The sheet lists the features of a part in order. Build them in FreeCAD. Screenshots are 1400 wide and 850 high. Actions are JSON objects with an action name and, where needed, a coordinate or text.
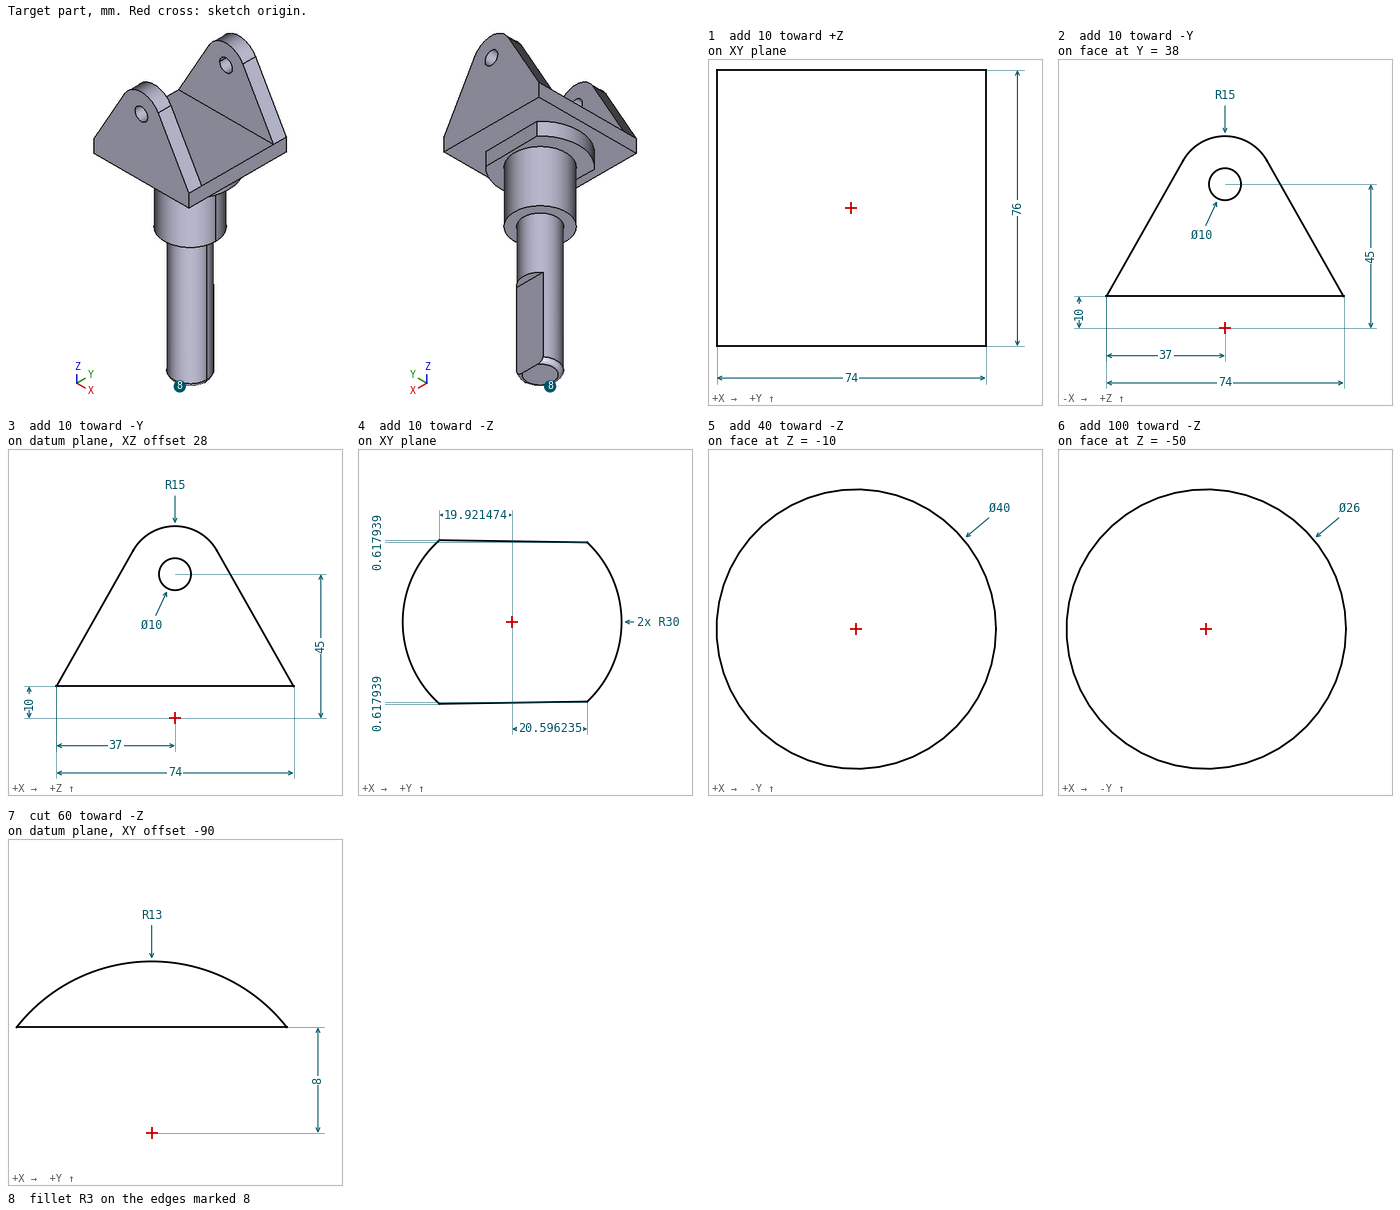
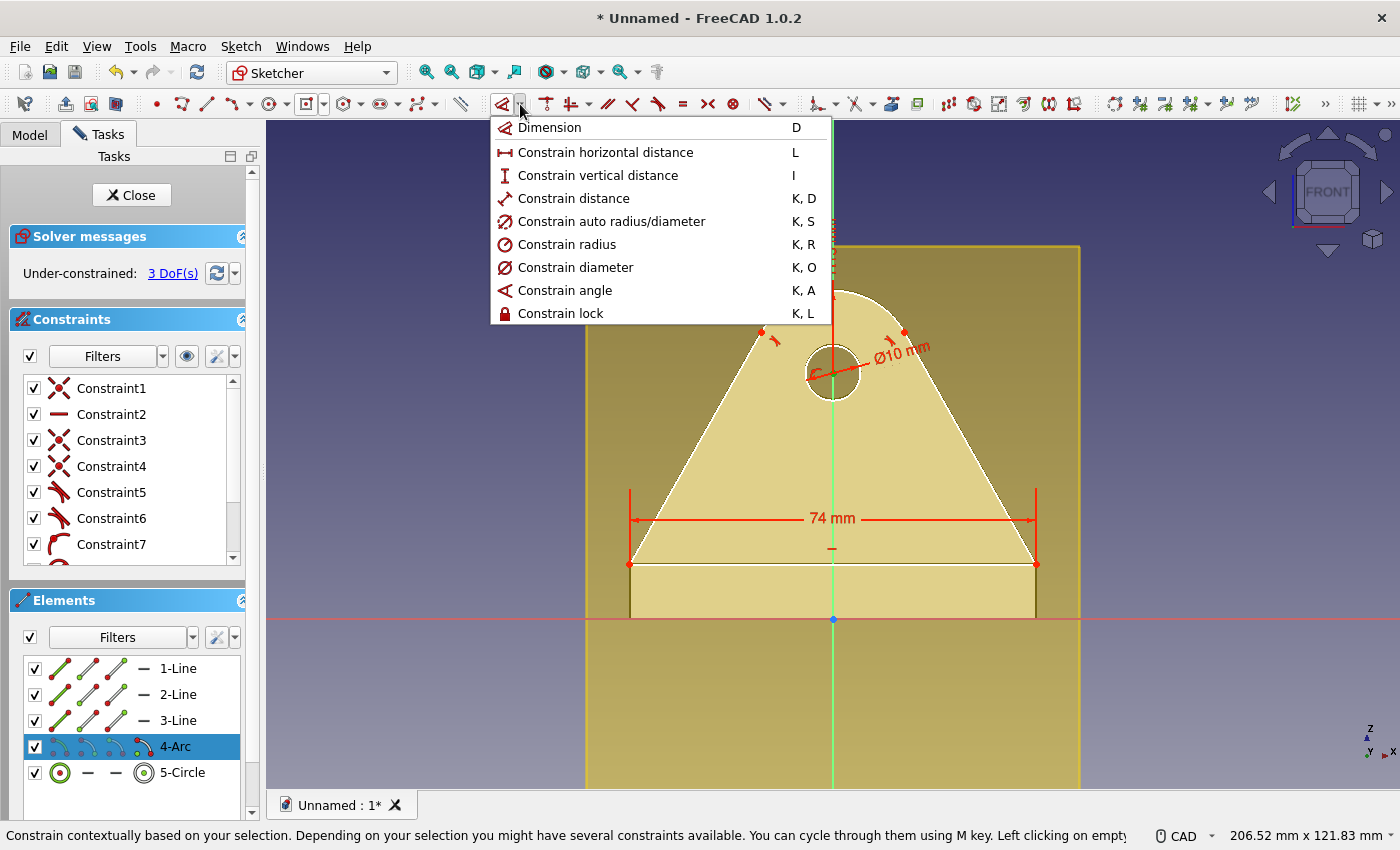
{"action": "left_click", "coordinate": [661, 176]}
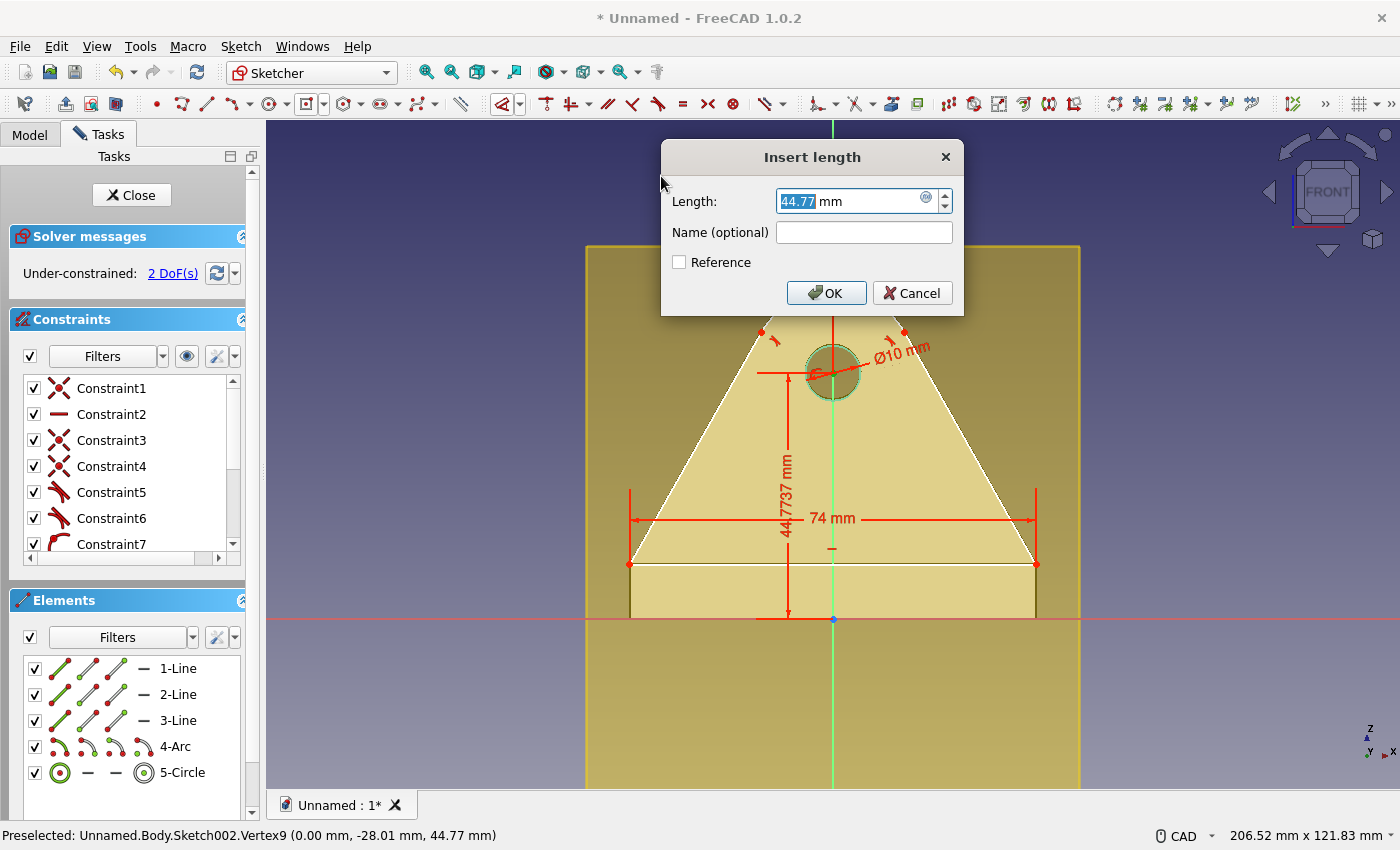
{"action": "type", "text": "45"}
{"action": "key", "text": "Return"}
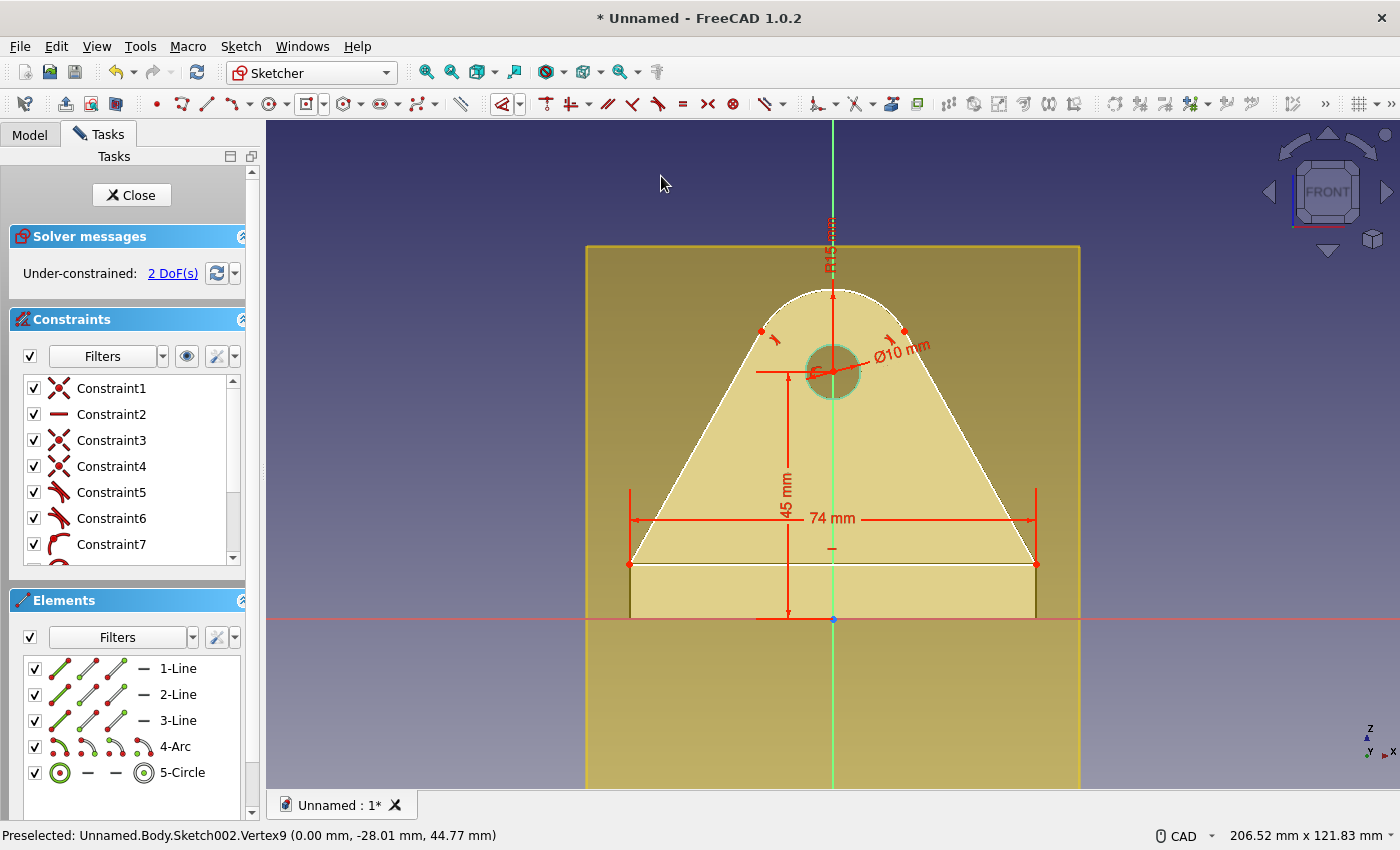
{"action": "left_click", "coordinate": [630, 565]}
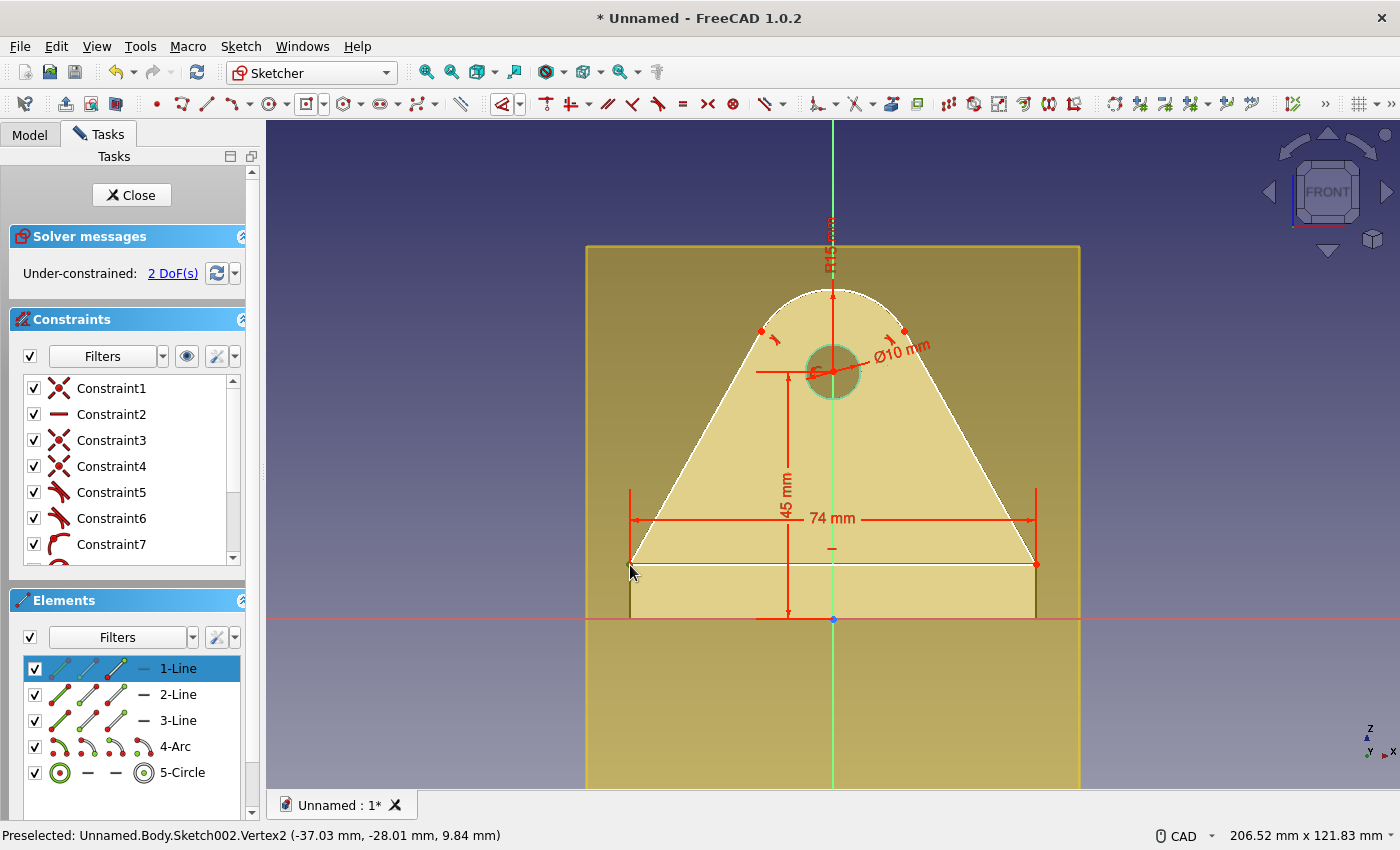
{"action": "left_click", "coordinate": [520, 104]}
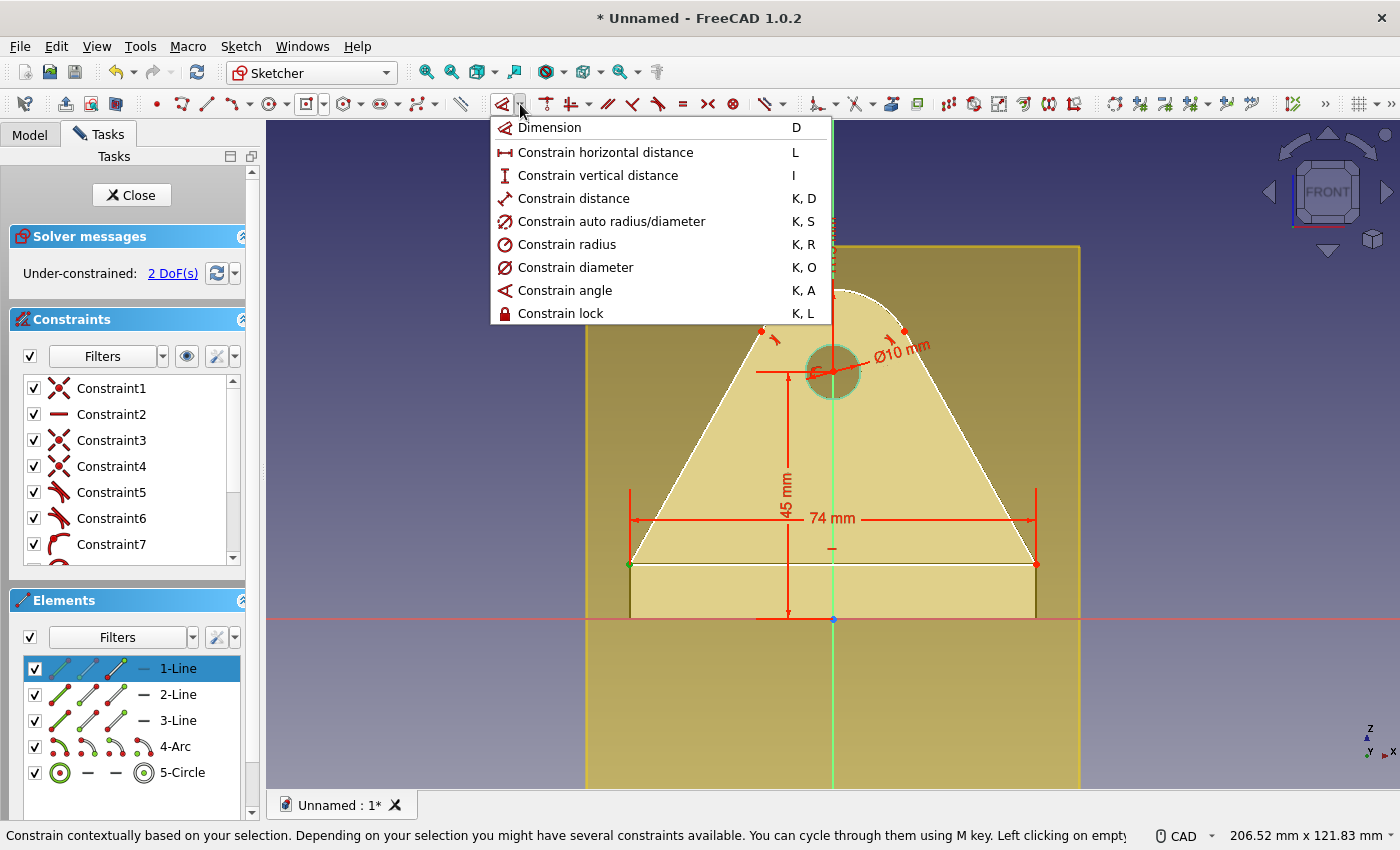
{"action": "left_click", "coordinate": [661, 152]}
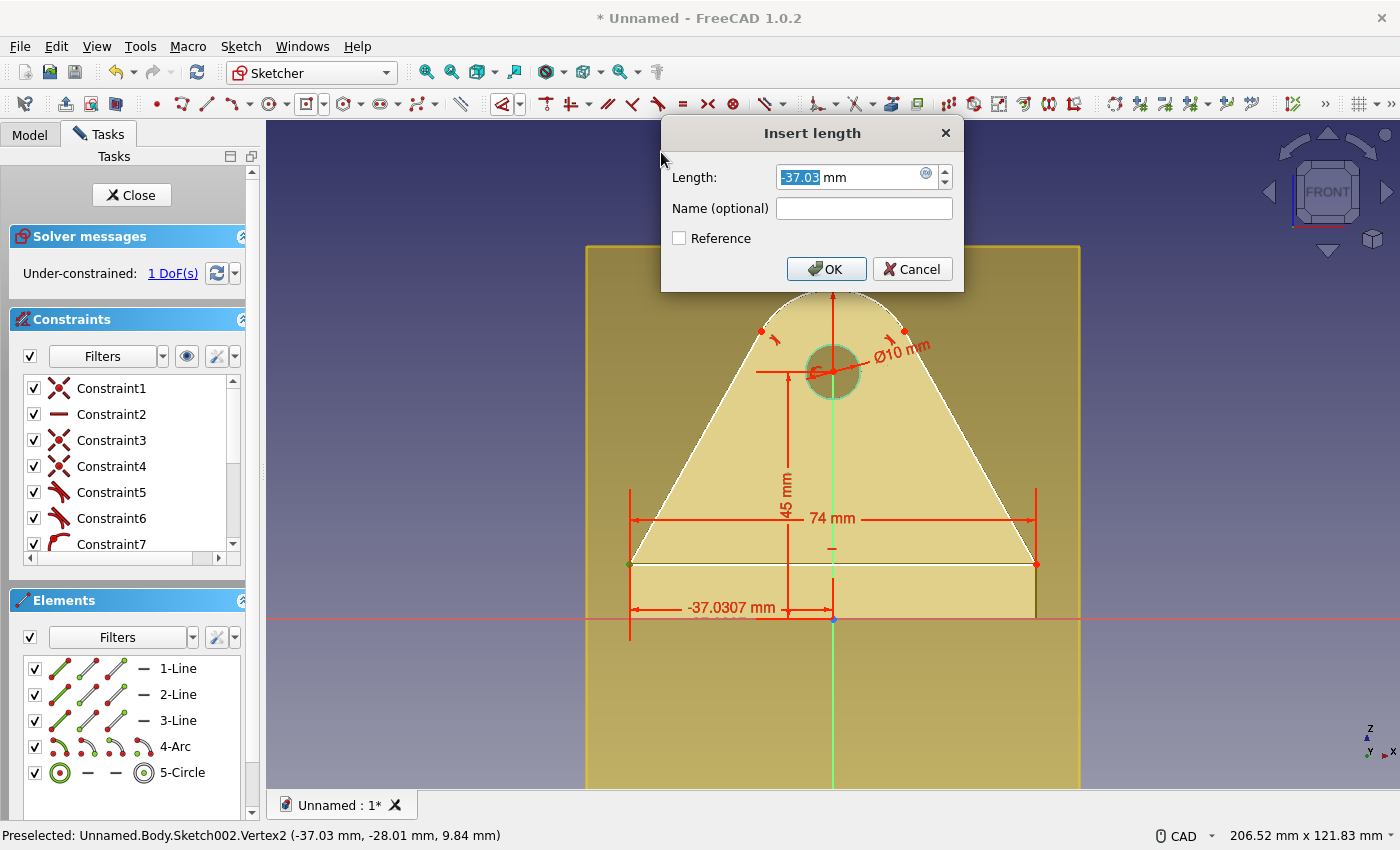
{"action": "type", "text": "-37"}
{"action": "key", "text": "Return"}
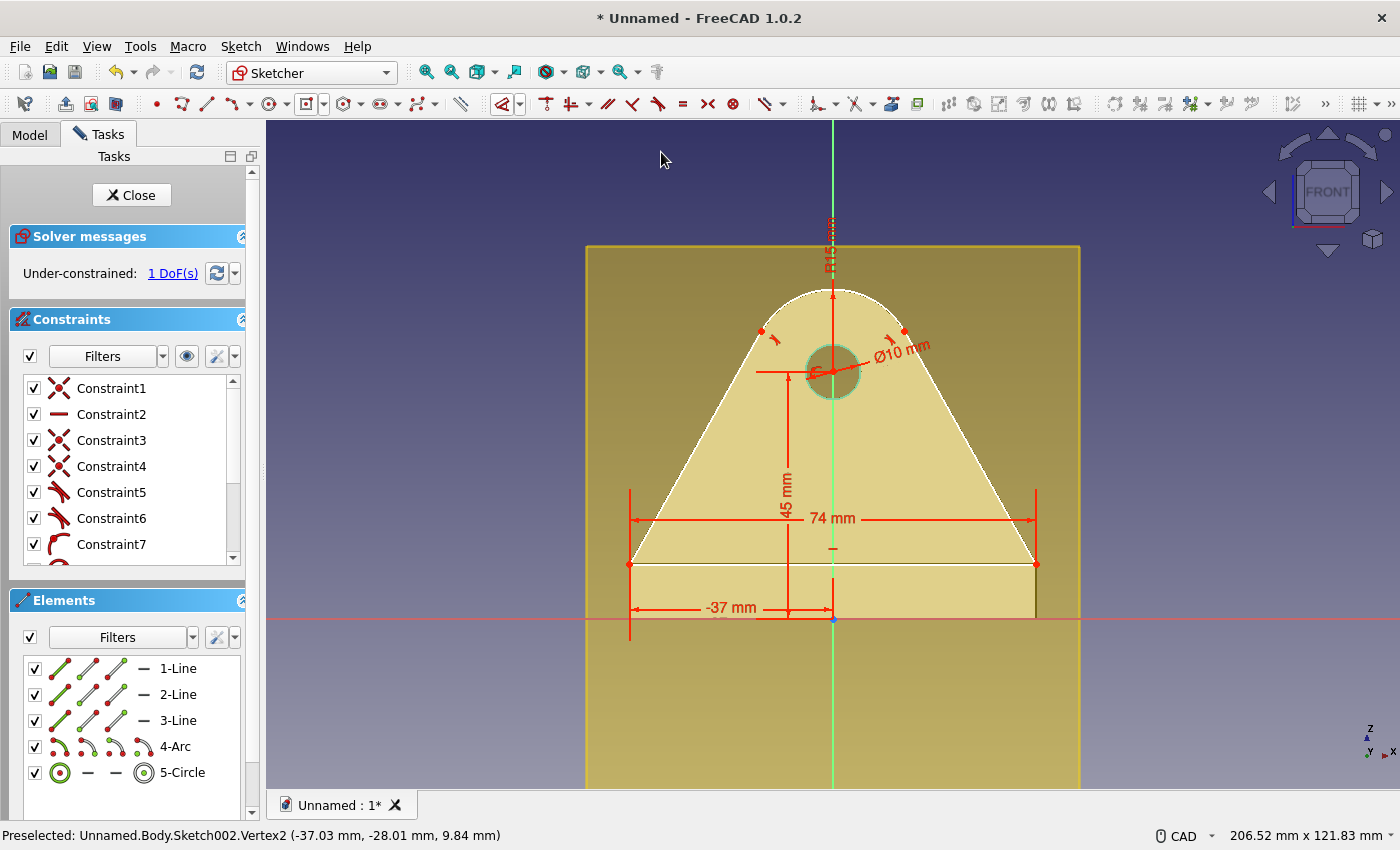
{"action": "left_click", "coordinate": [630, 565]}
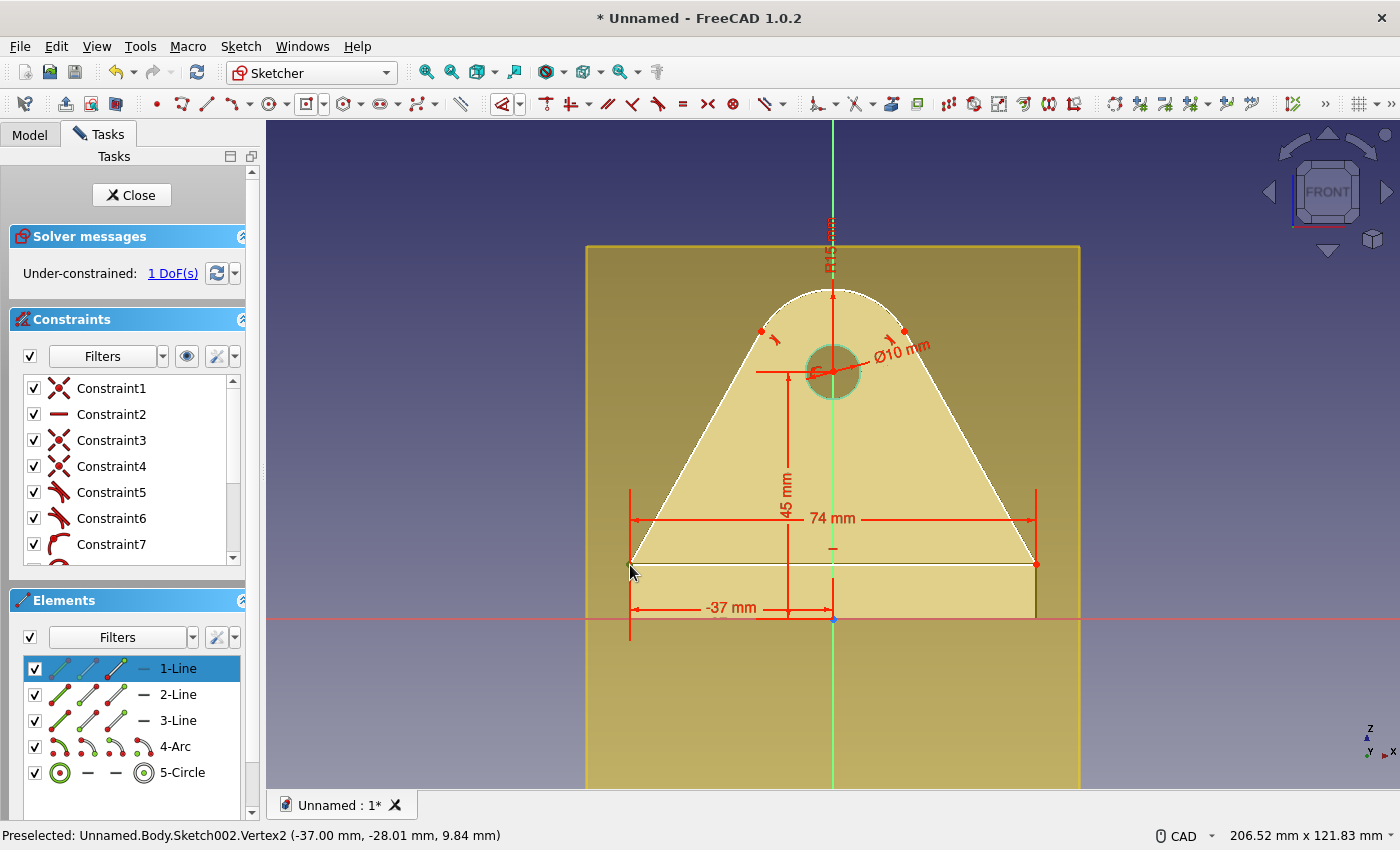
{"action": "left_click", "coordinate": [520, 104]}